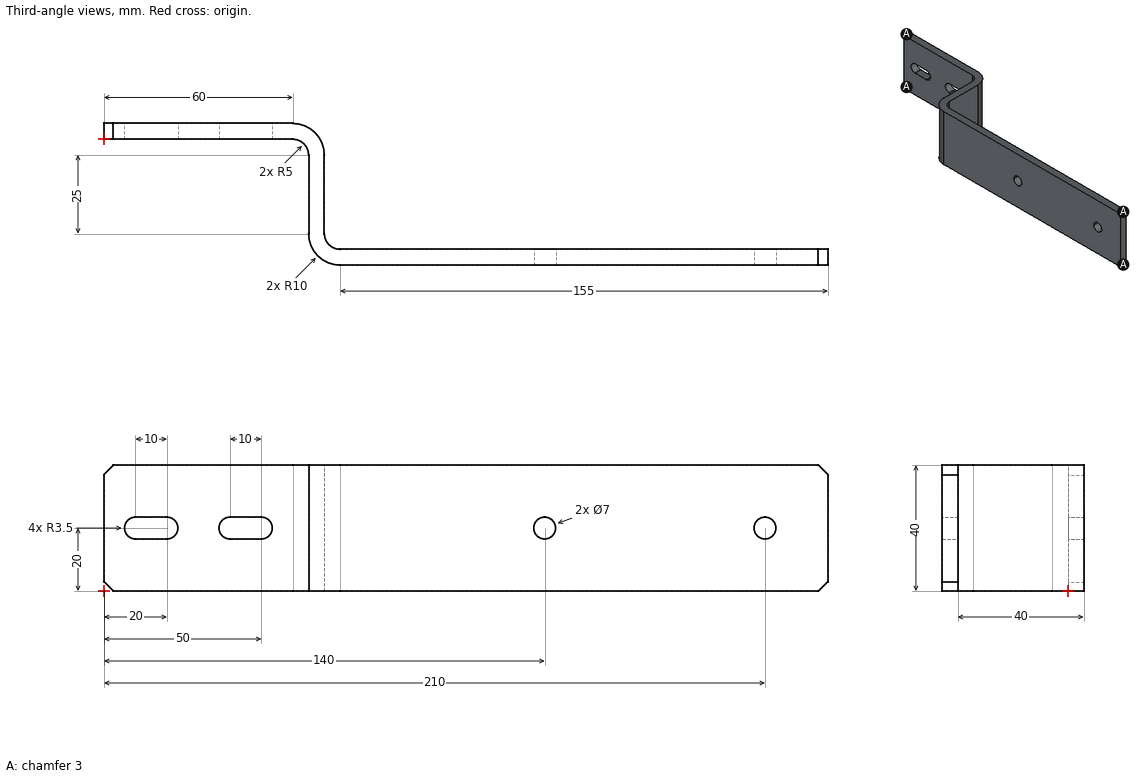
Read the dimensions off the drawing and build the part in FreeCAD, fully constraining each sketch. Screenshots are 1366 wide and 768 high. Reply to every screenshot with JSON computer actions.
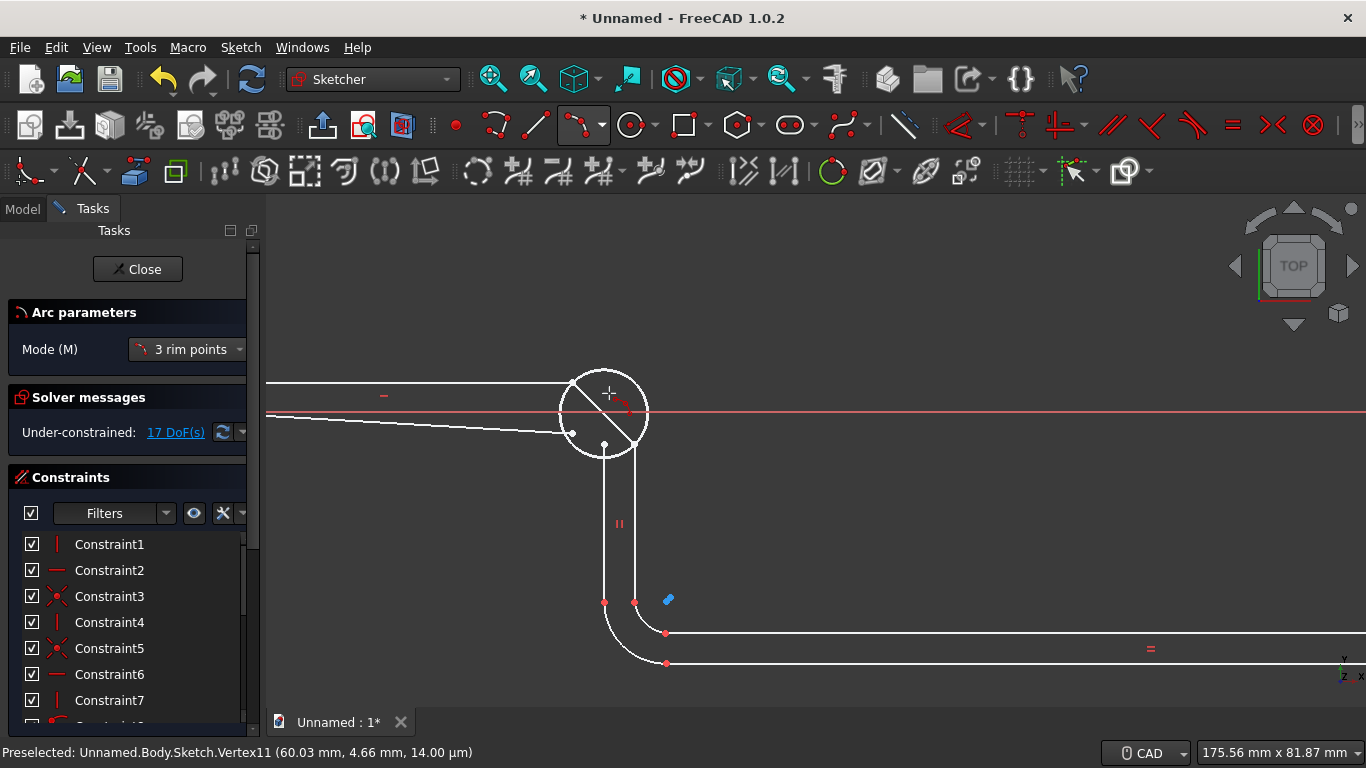
{"action": "left_click", "coordinate": [609, 393]}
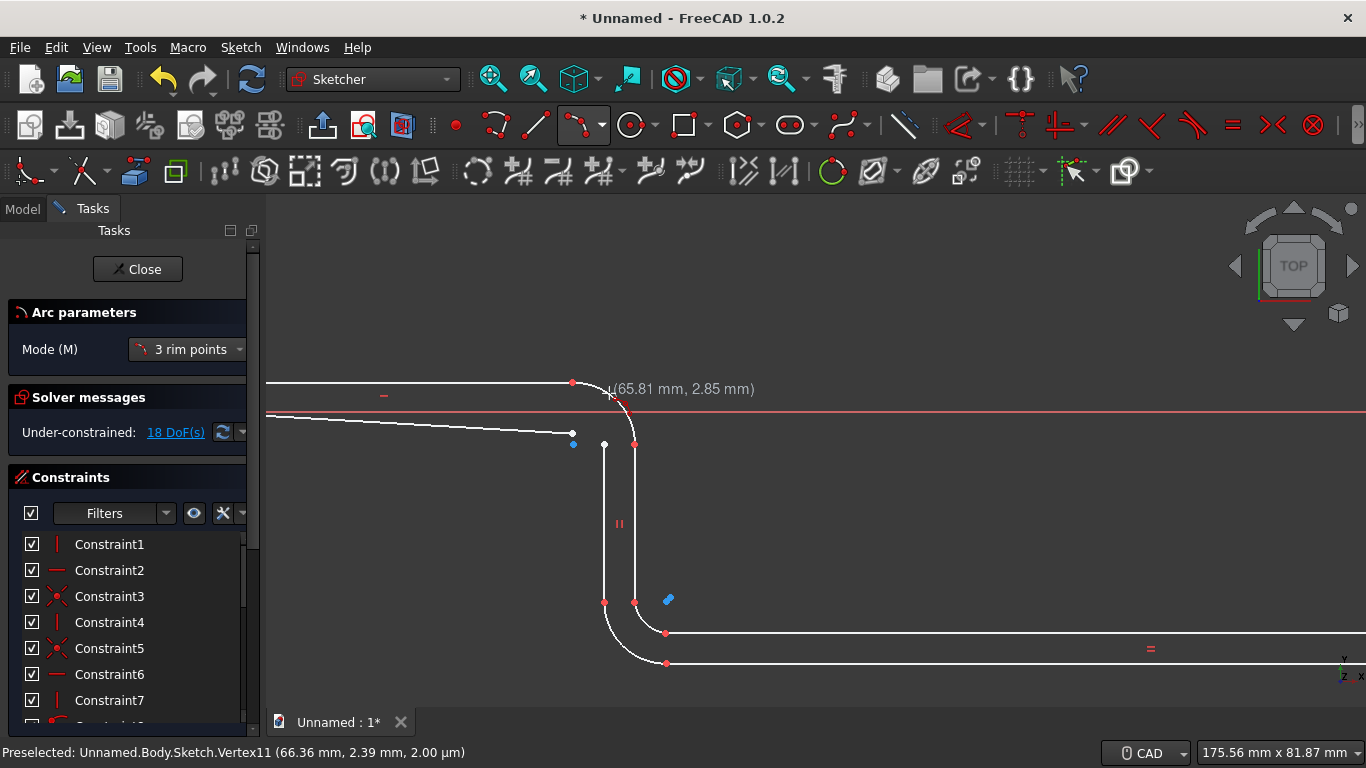
{"action": "left_click", "coordinate": [573, 434]}
{"action": "left_click", "coordinate": [604, 444]}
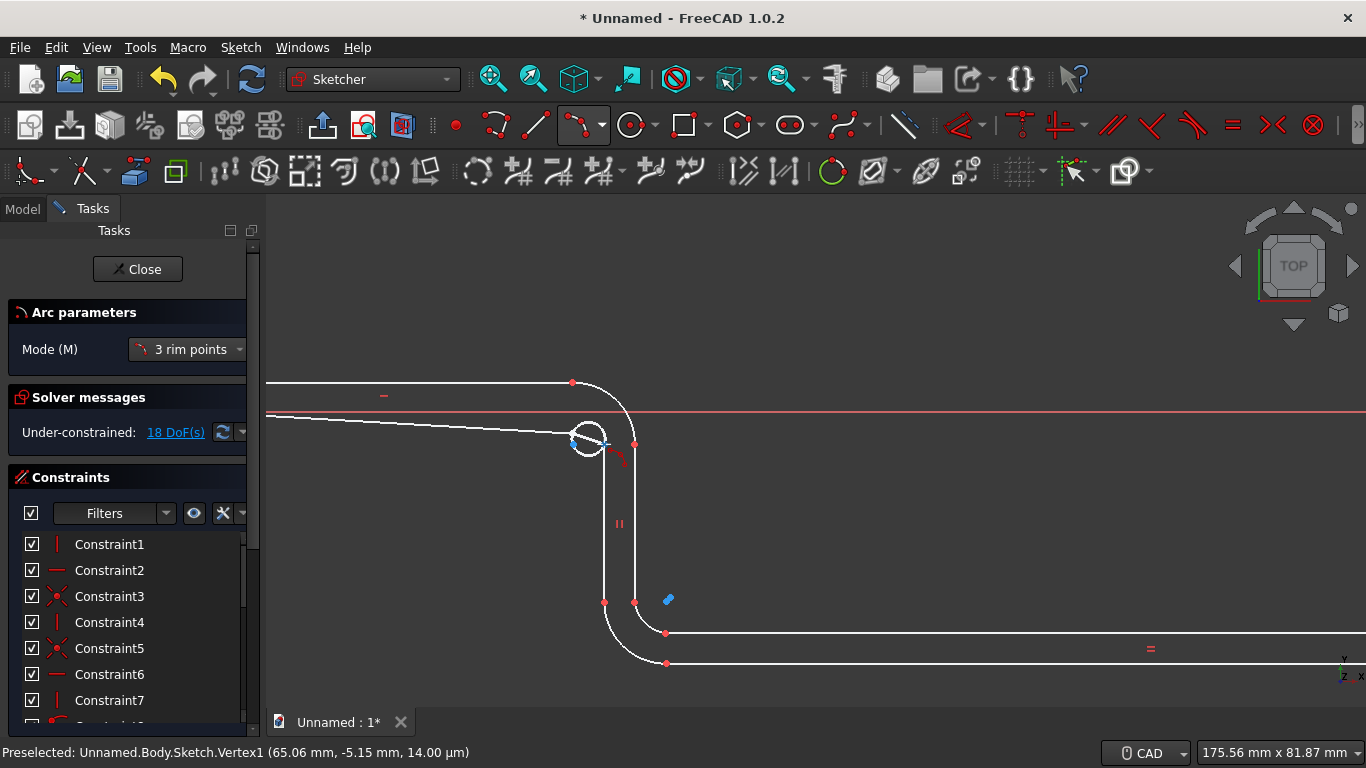
{"action": "scroll", "coordinate": [595, 421], "scroll_direction": "up", "scroll_amount": 3}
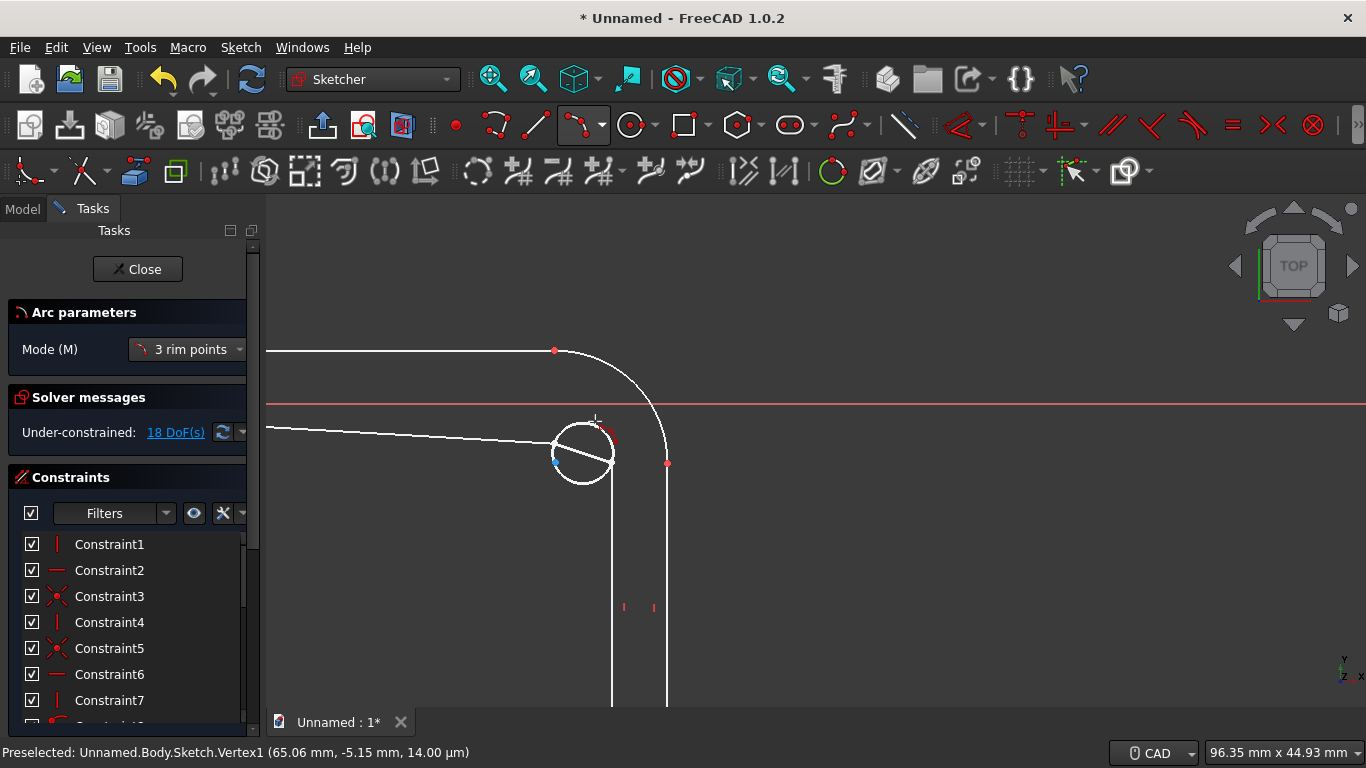
{"action": "left_click", "coordinate": [594, 421]}
{"action": "key", "text": "Escape"}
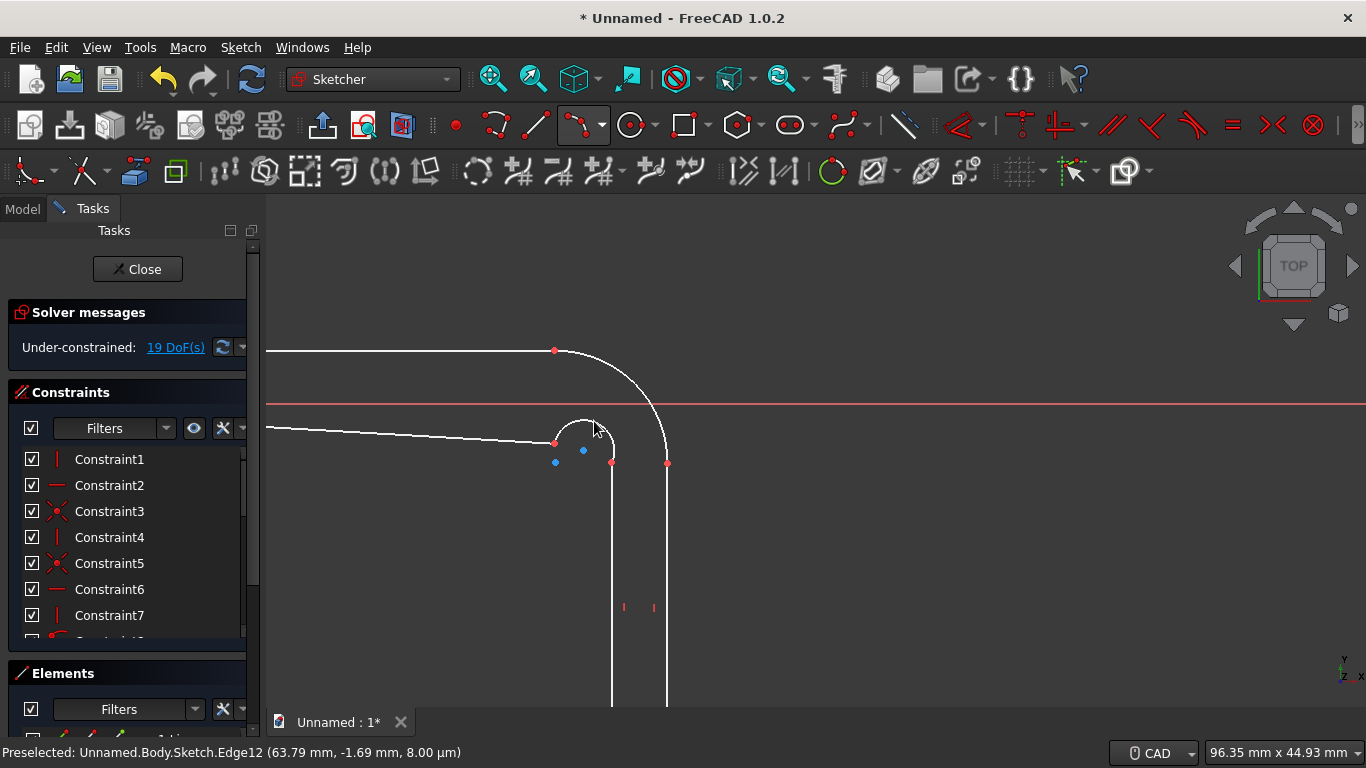
{"action": "scroll", "coordinate": [605, 400], "scroll_direction": "down", "scroll_amount": 7}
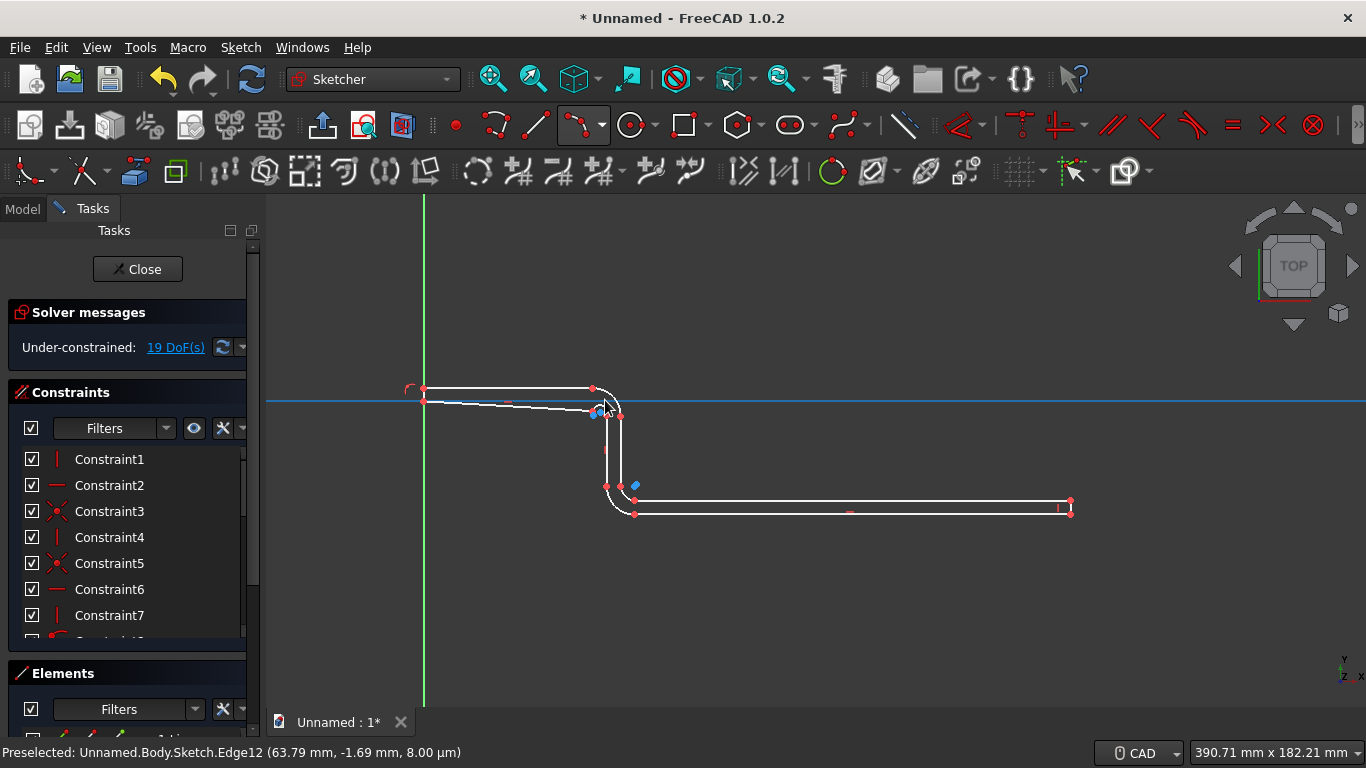
{"action": "left_click", "coordinate": [607, 437]}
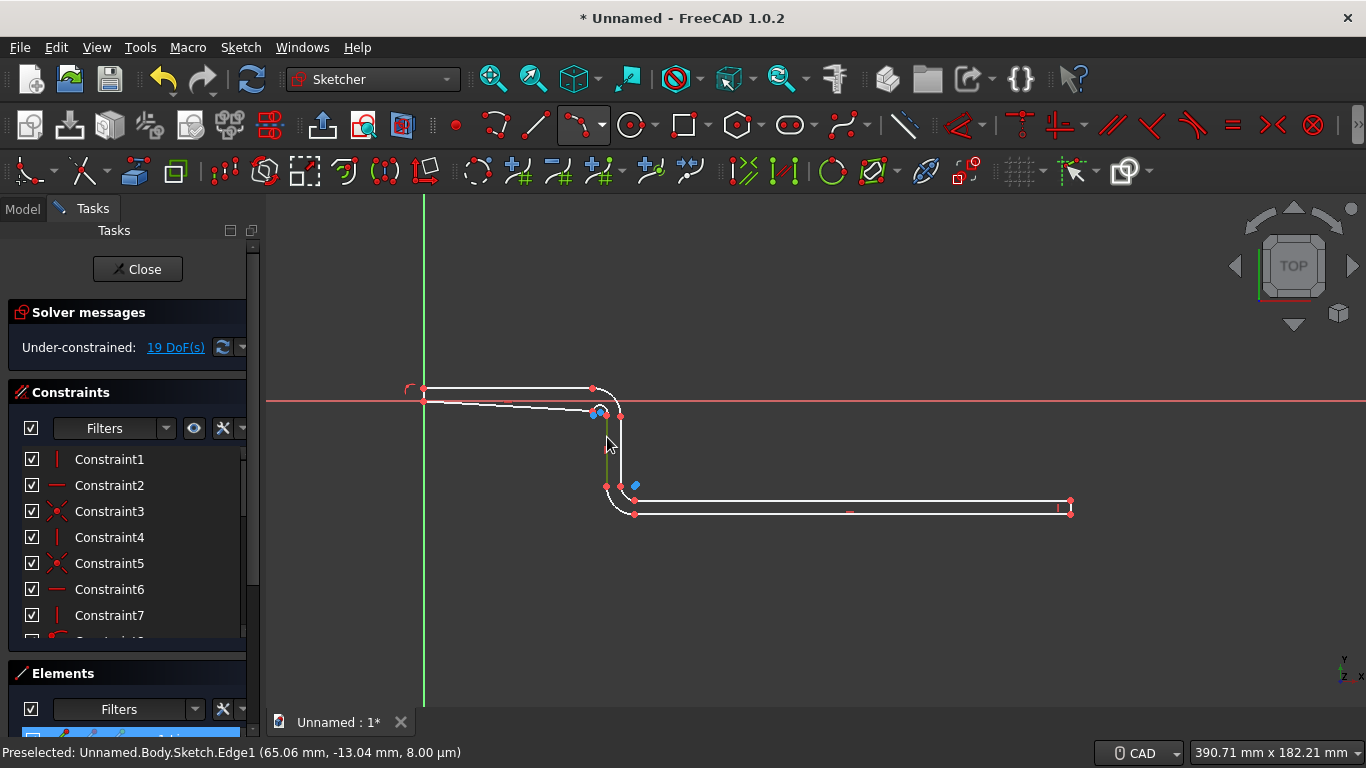
{"action": "left_click", "coordinate": [610, 499]}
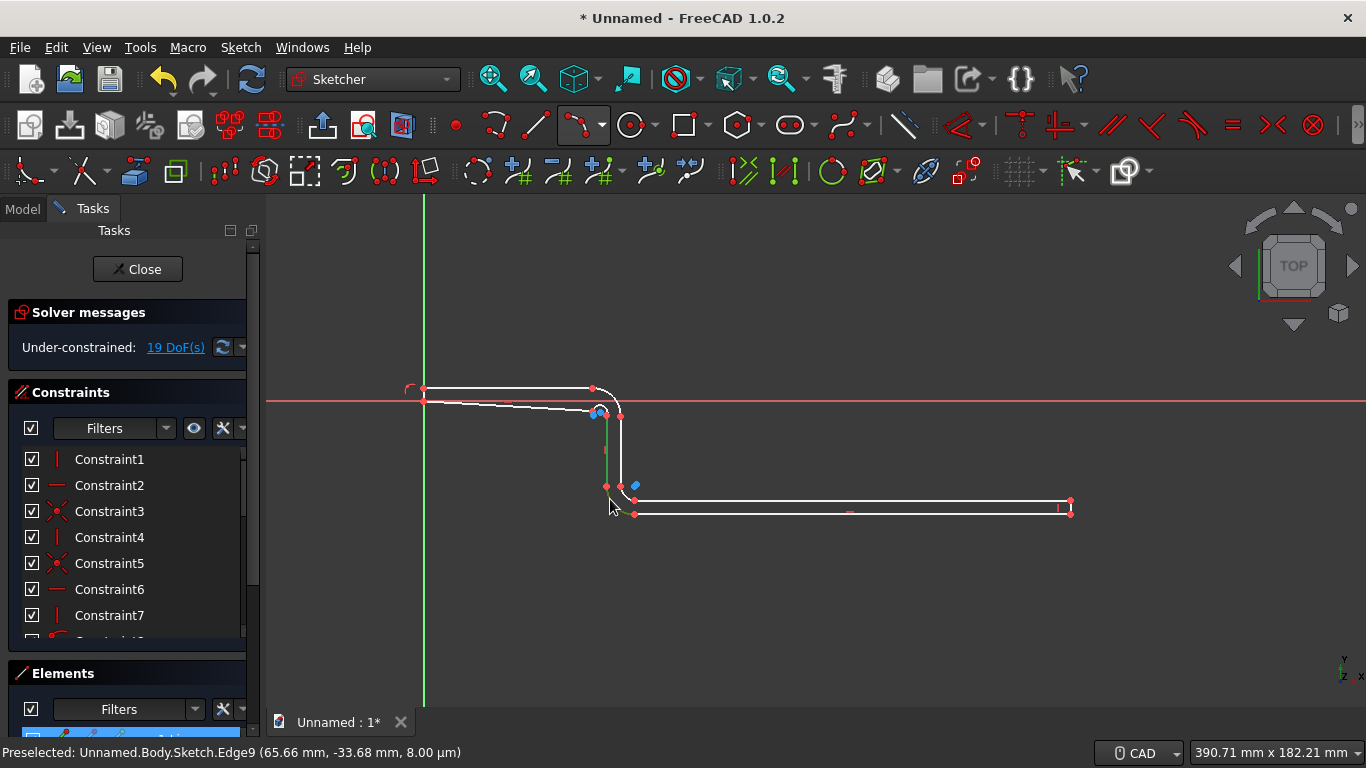
{"action": "left_click", "coordinate": [1194, 126]}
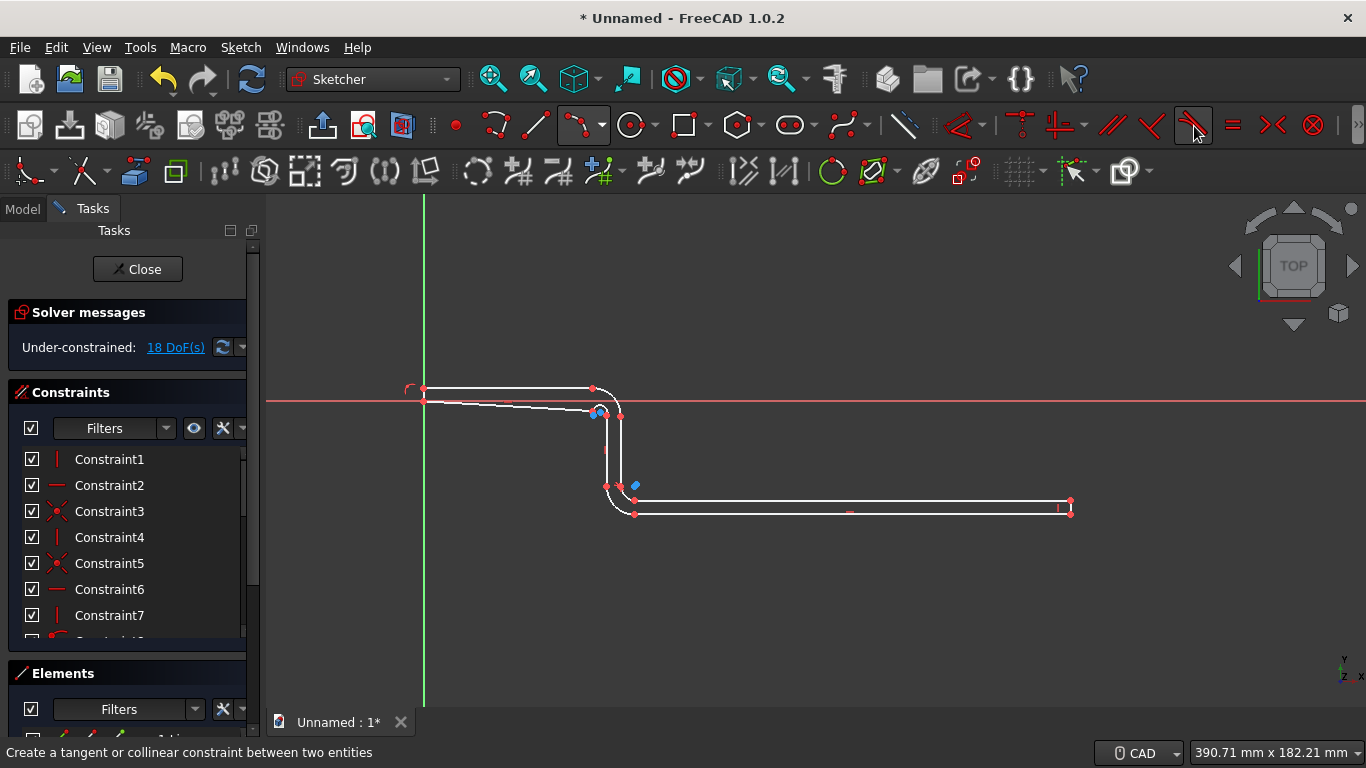
{"action": "left_click", "coordinate": [607, 437]}